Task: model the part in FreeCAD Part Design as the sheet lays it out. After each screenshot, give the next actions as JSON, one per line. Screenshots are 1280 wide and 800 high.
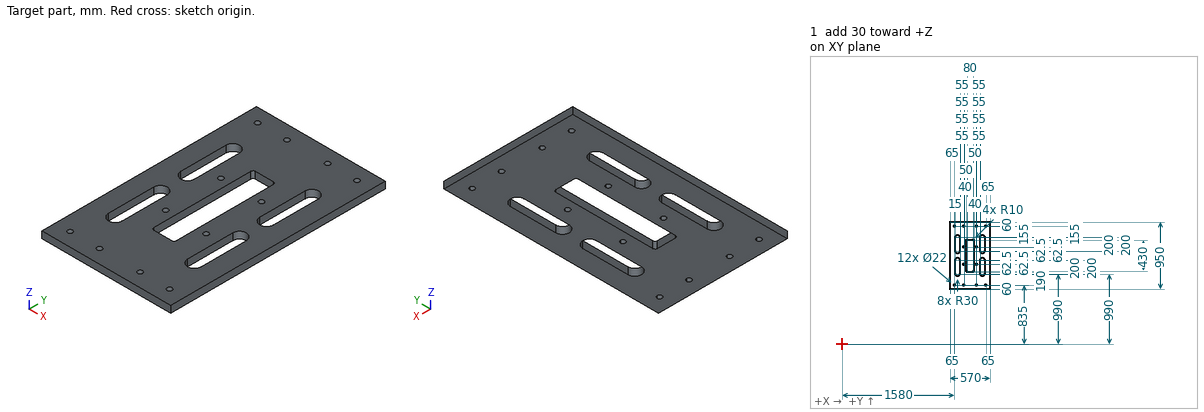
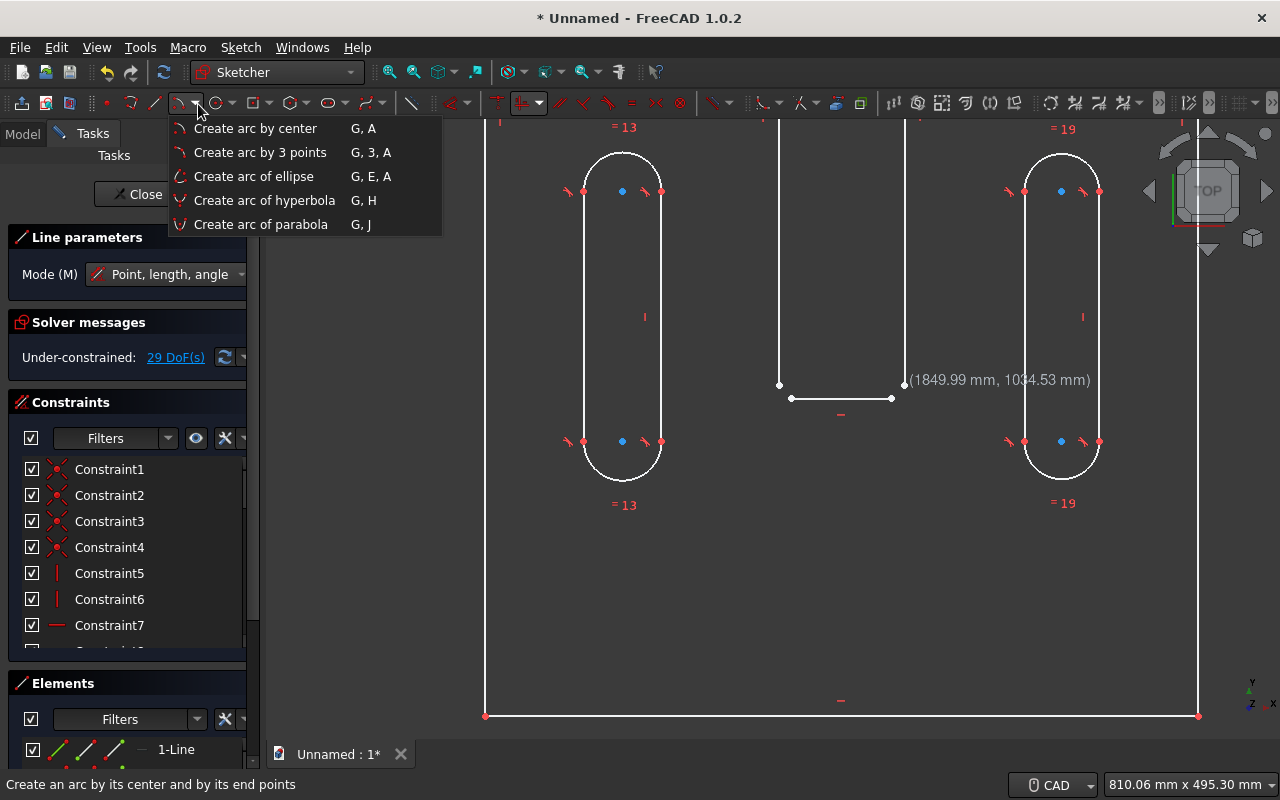
{"action": "left_click", "coordinate": [306, 152]}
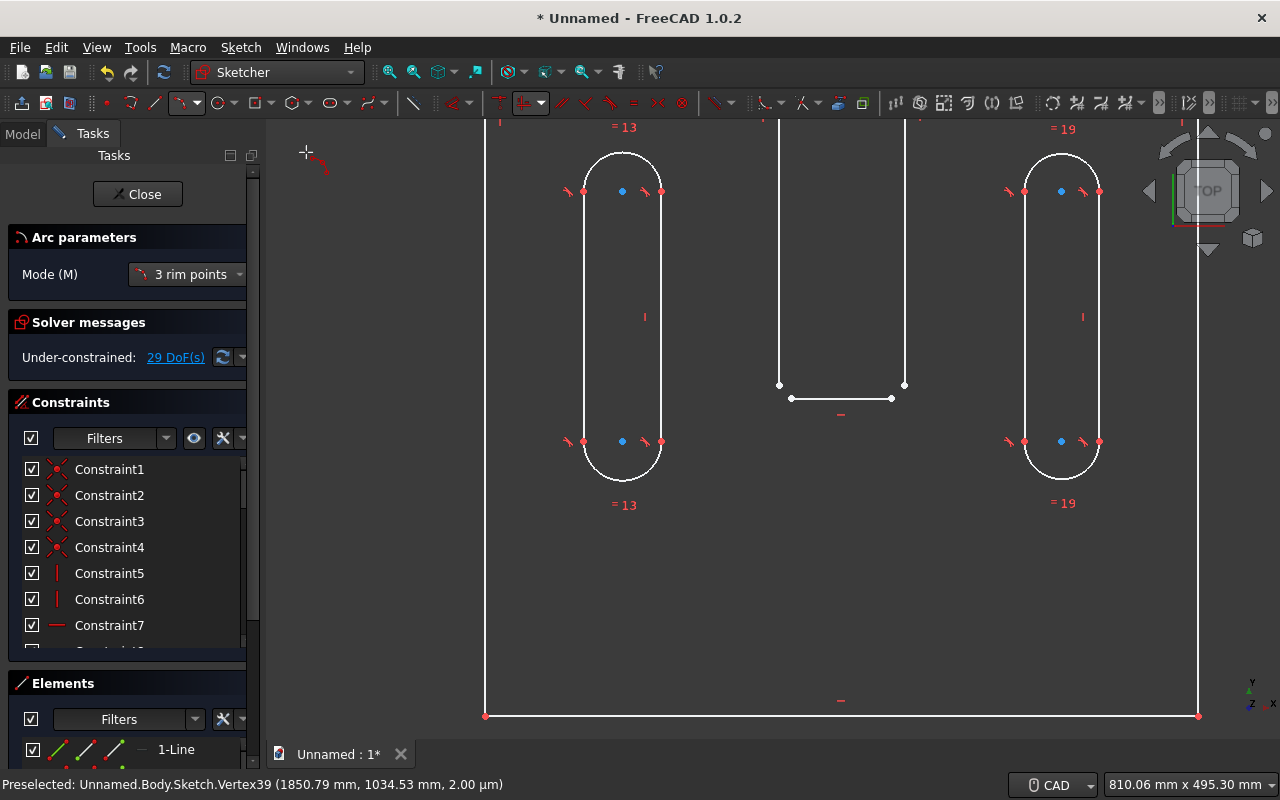
{"action": "left_click", "coordinate": [792, 399]}
{"action": "left_click", "coordinate": [779, 385]}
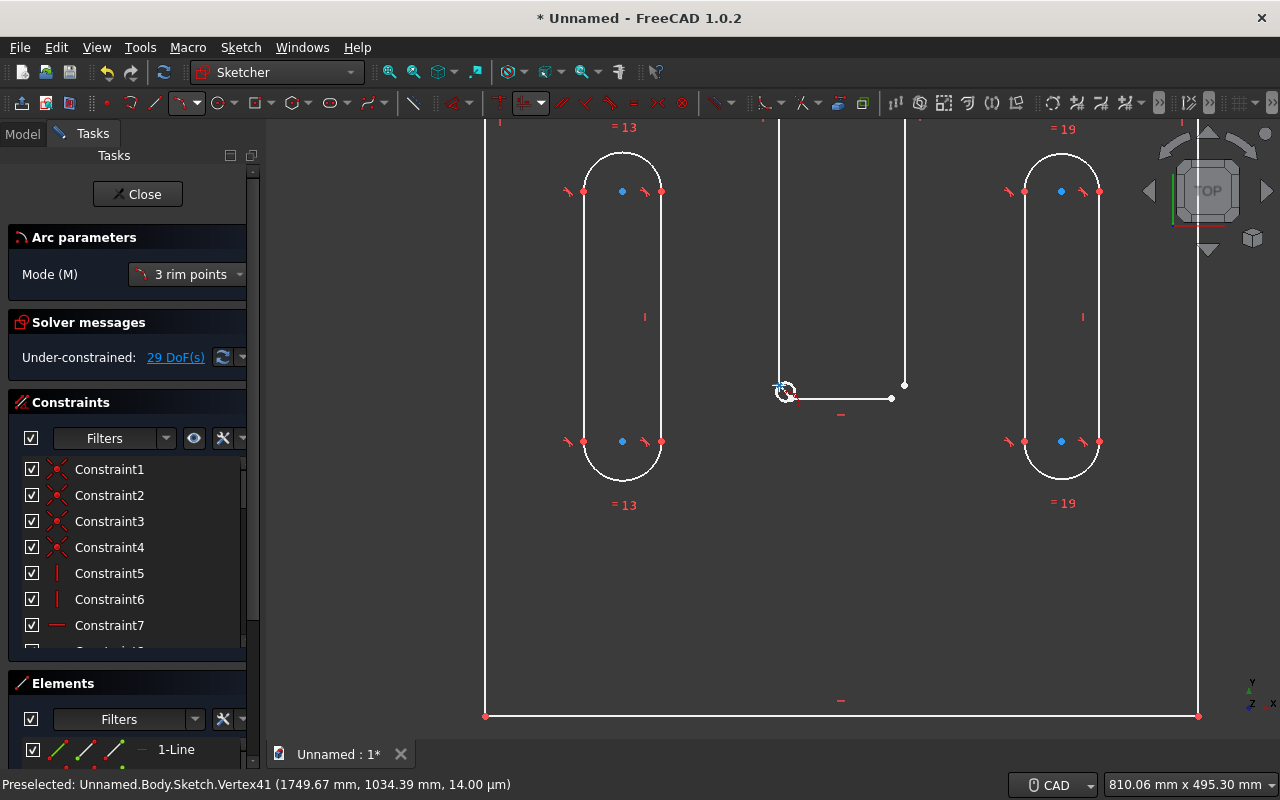
{"action": "scroll", "coordinate": [784, 393], "scroll_direction": "up", "scroll_amount": 8}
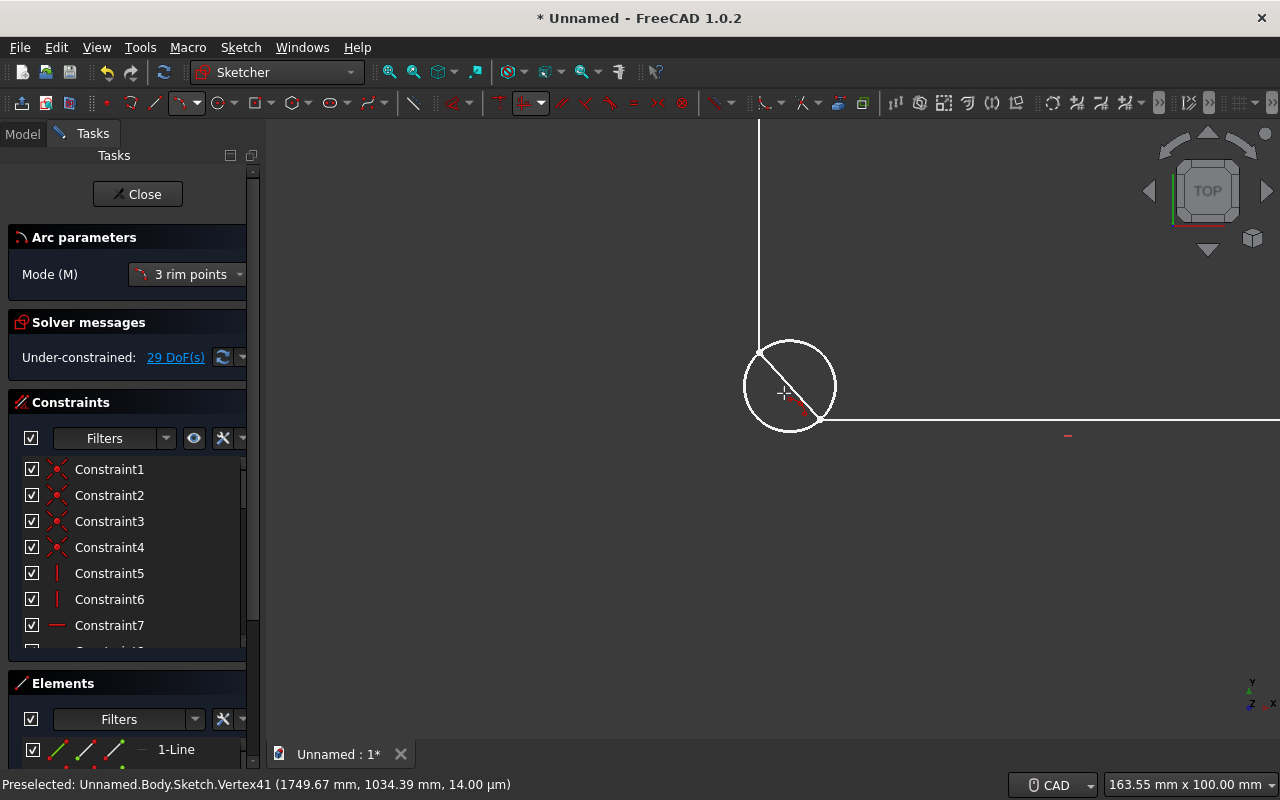
{"action": "left_click", "coordinate": [780, 393]}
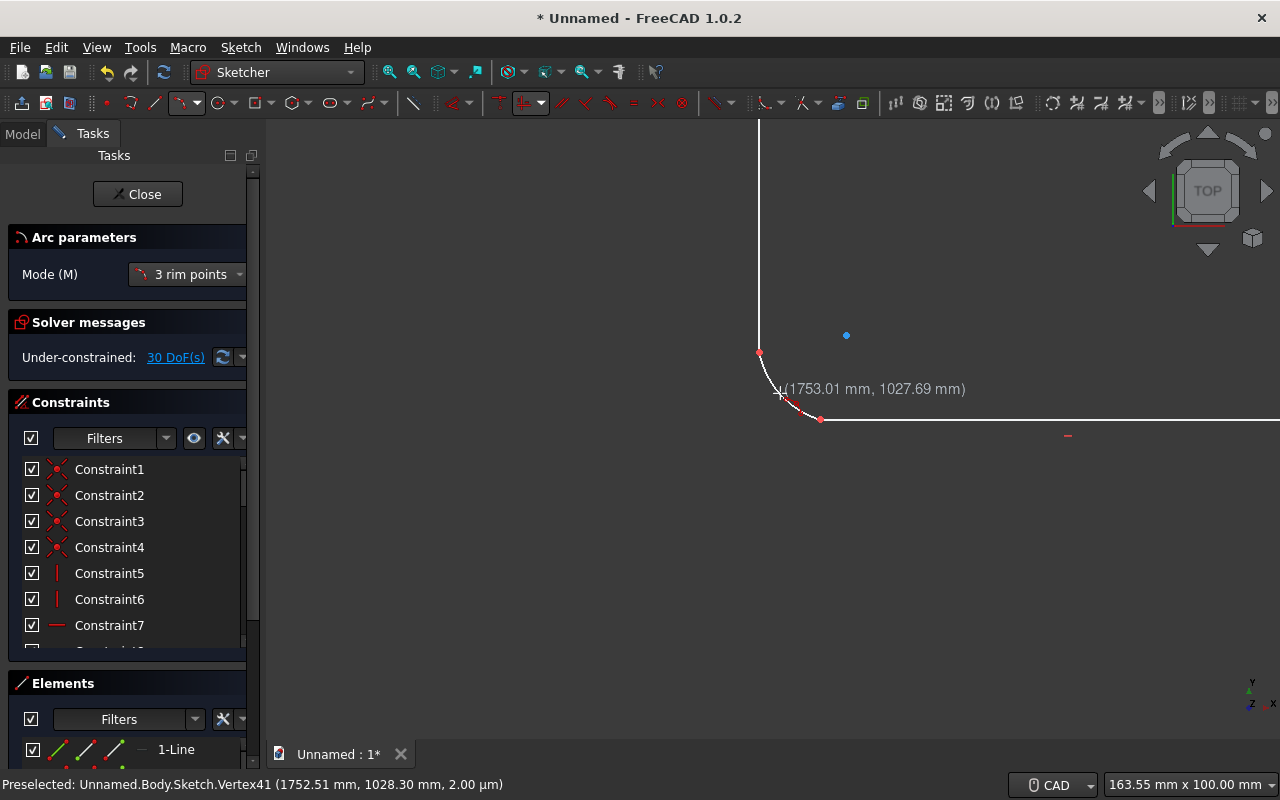
{"action": "scroll", "coordinate": [888, 387], "scroll_direction": "down", "scroll_amount": 16}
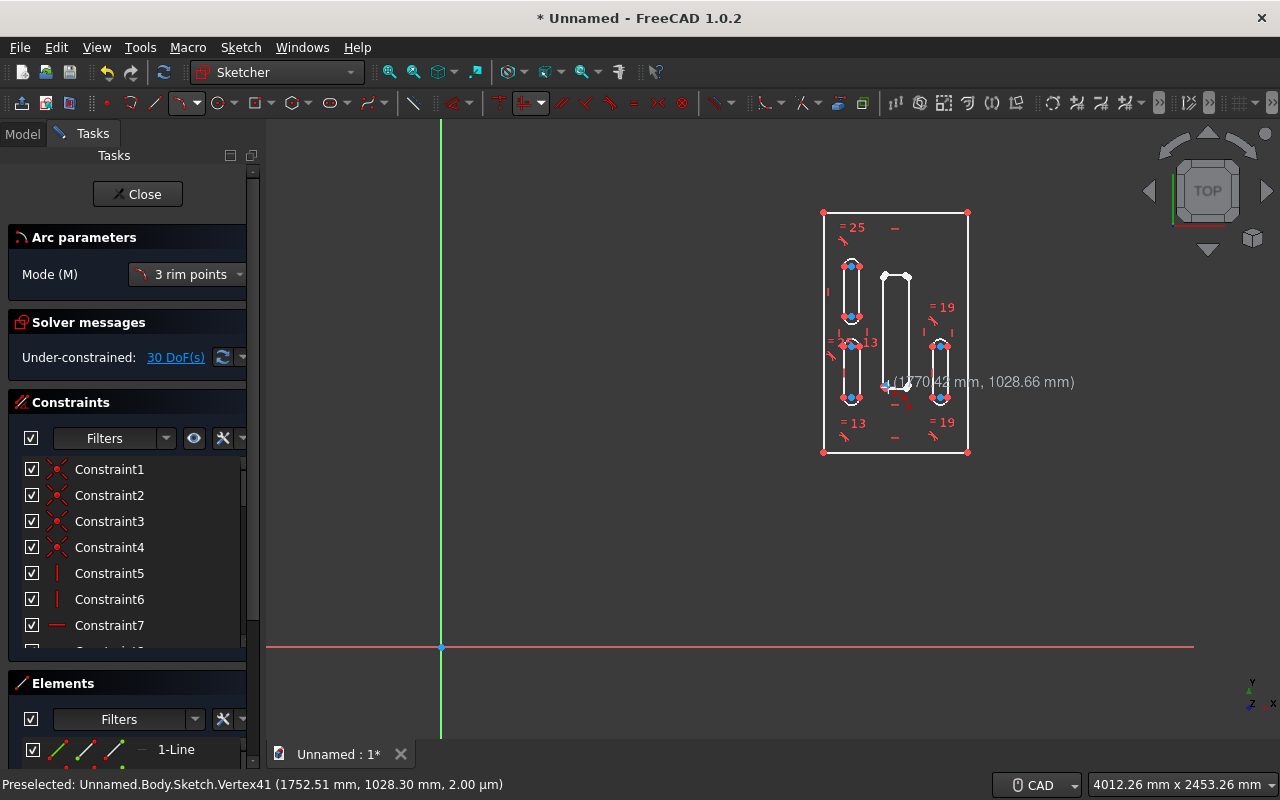
{"action": "scroll", "coordinate": [883, 277], "scroll_direction": "up", "scroll_amount": 8}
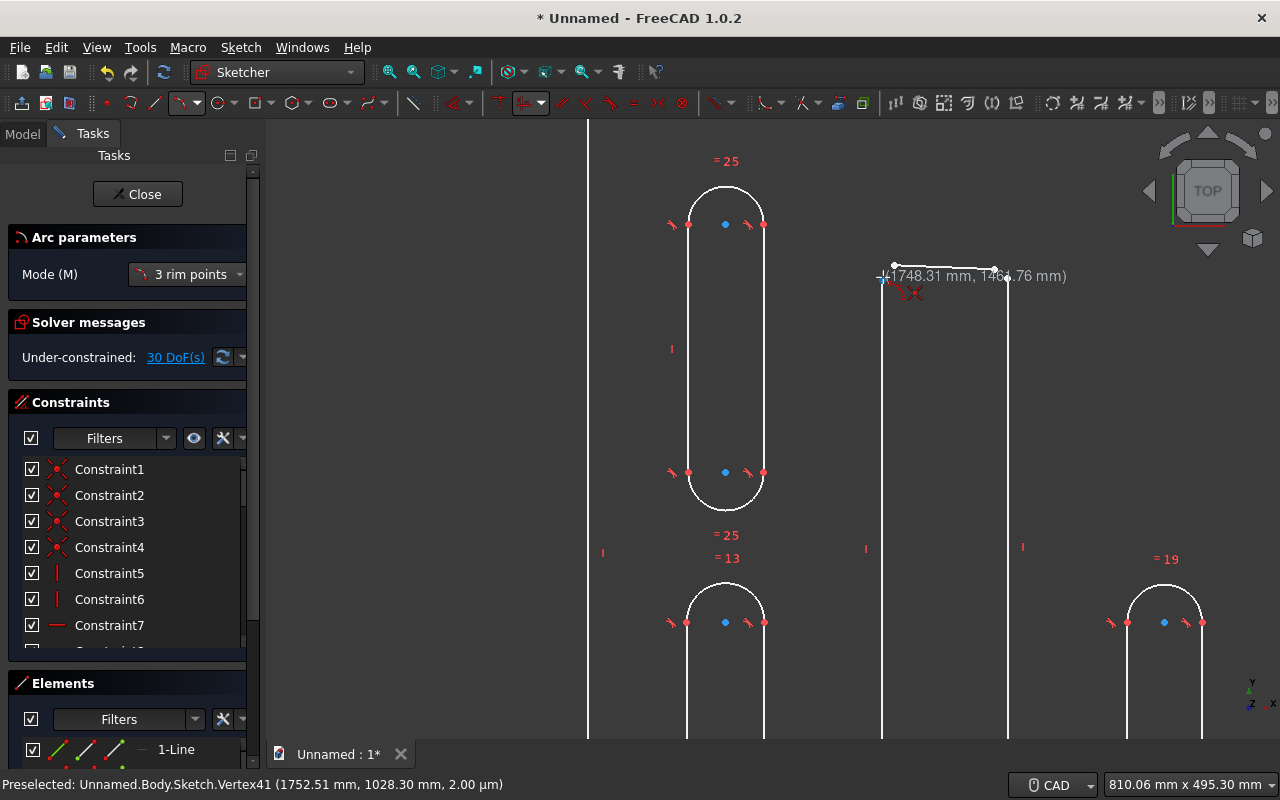
{"action": "left_click", "coordinate": [882, 280]}
{"action": "left_click", "coordinate": [895, 265]}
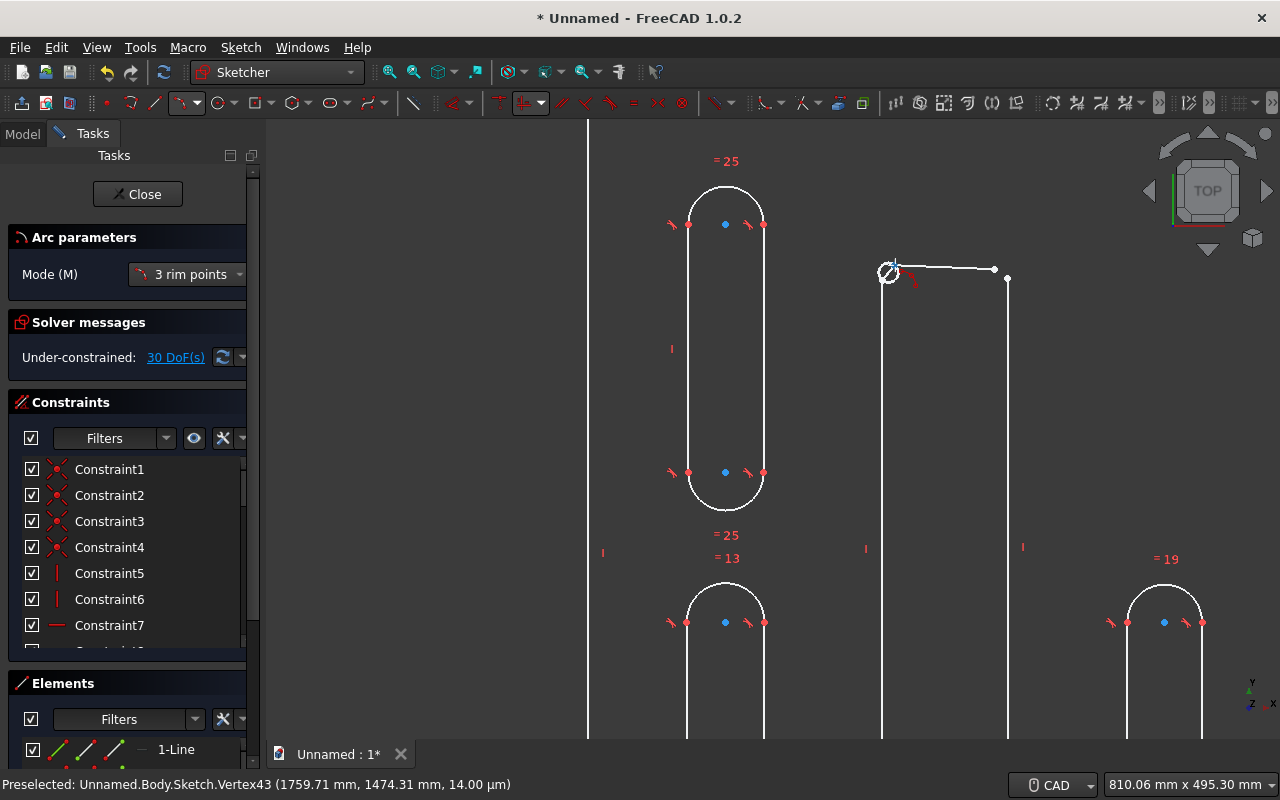
{"action": "scroll", "coordinate": [886, 268], "scroll_direction": "up", "scroll_amount": 8}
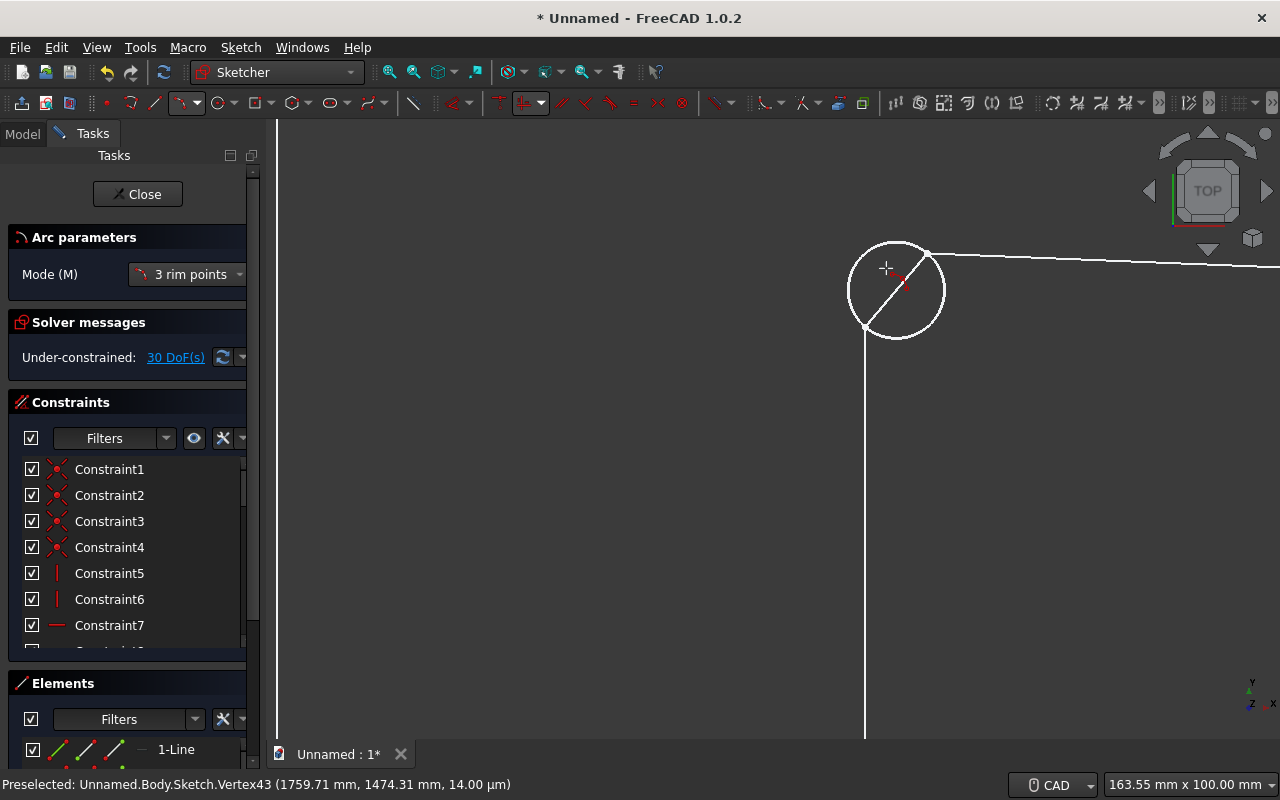
{"action": "left_click", "coordinate": [885, 267]}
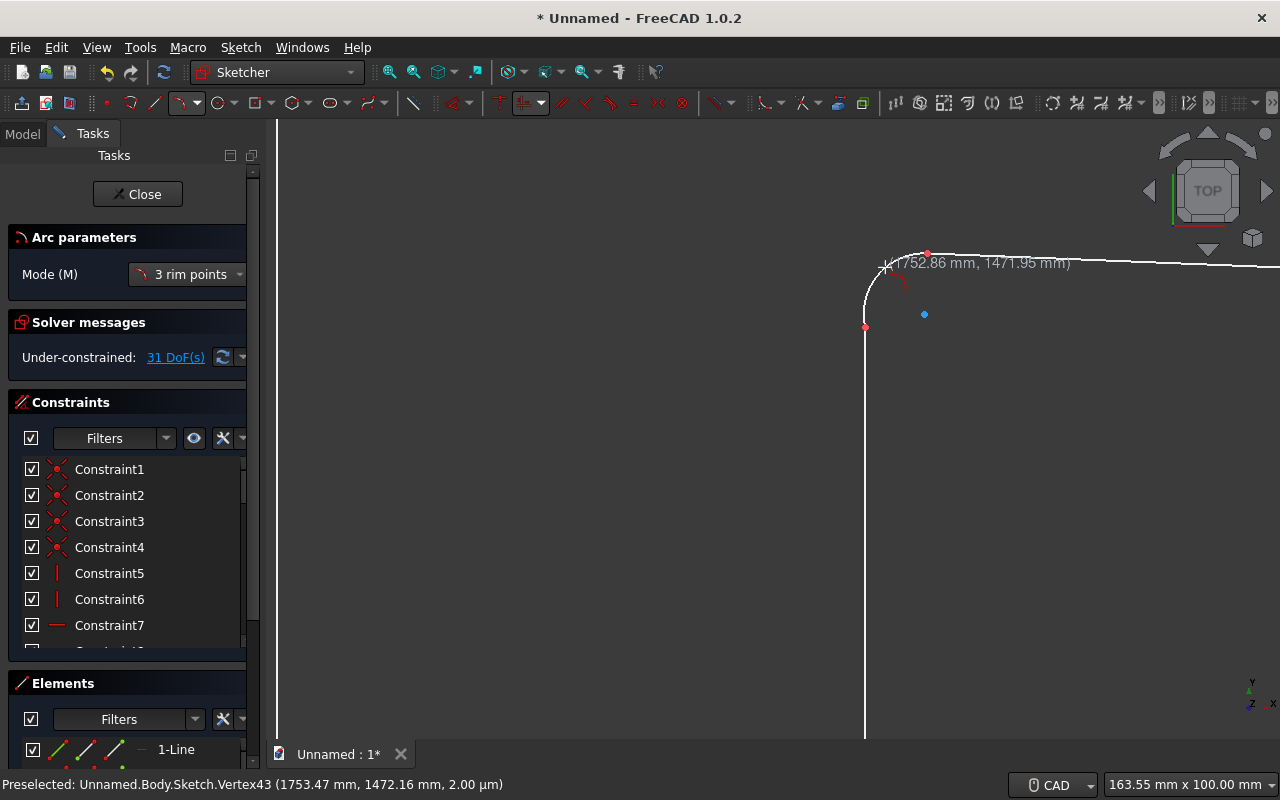
{"action": "scroll", "coordinate": [884, 275], "scroll_direction": "down", "scroll_amount": 16}